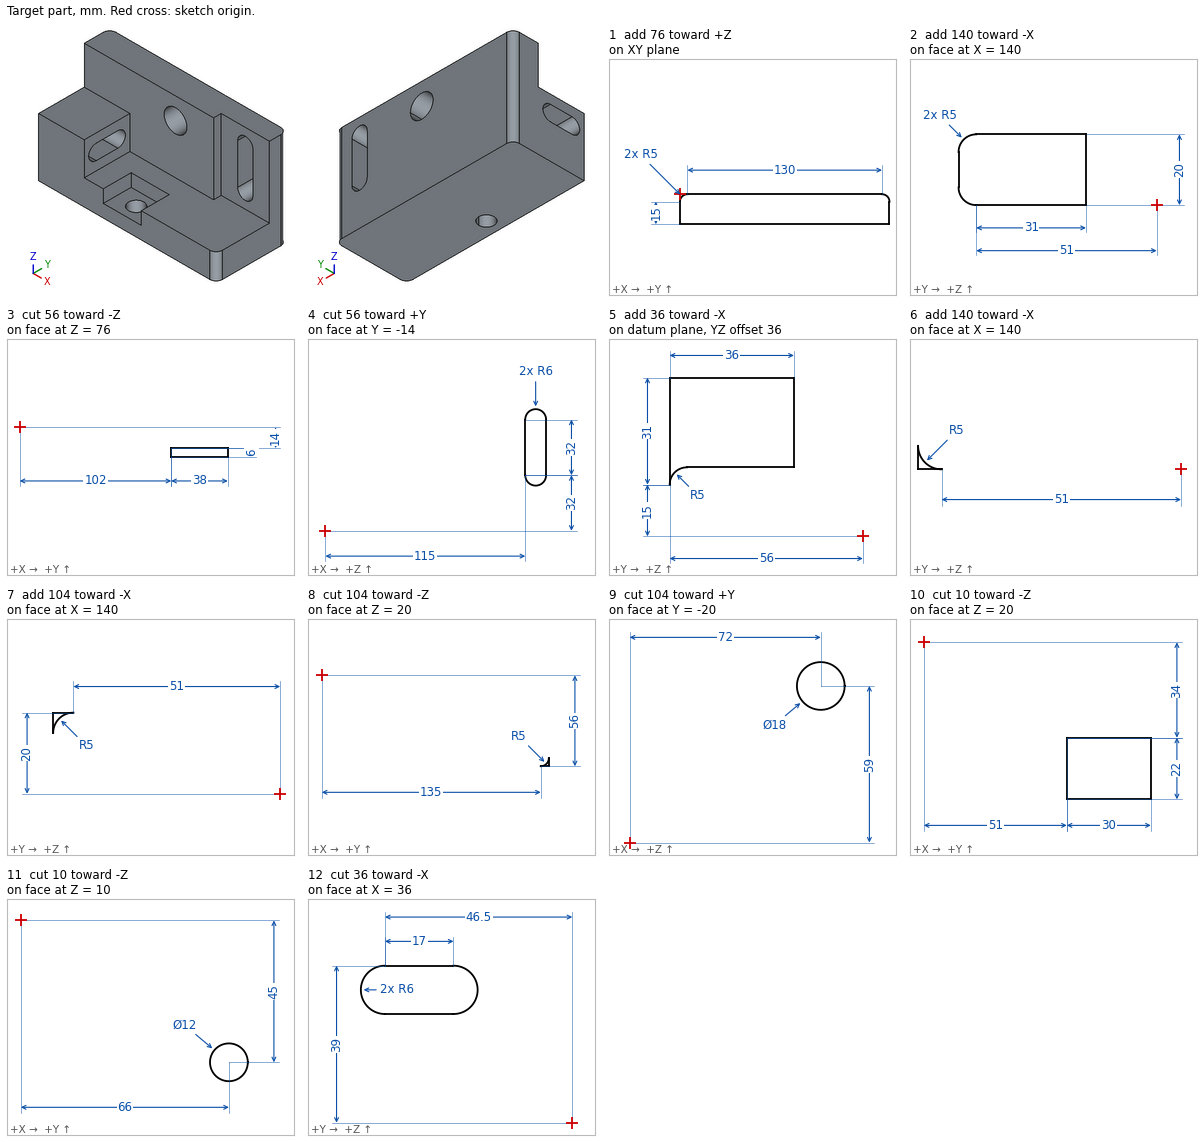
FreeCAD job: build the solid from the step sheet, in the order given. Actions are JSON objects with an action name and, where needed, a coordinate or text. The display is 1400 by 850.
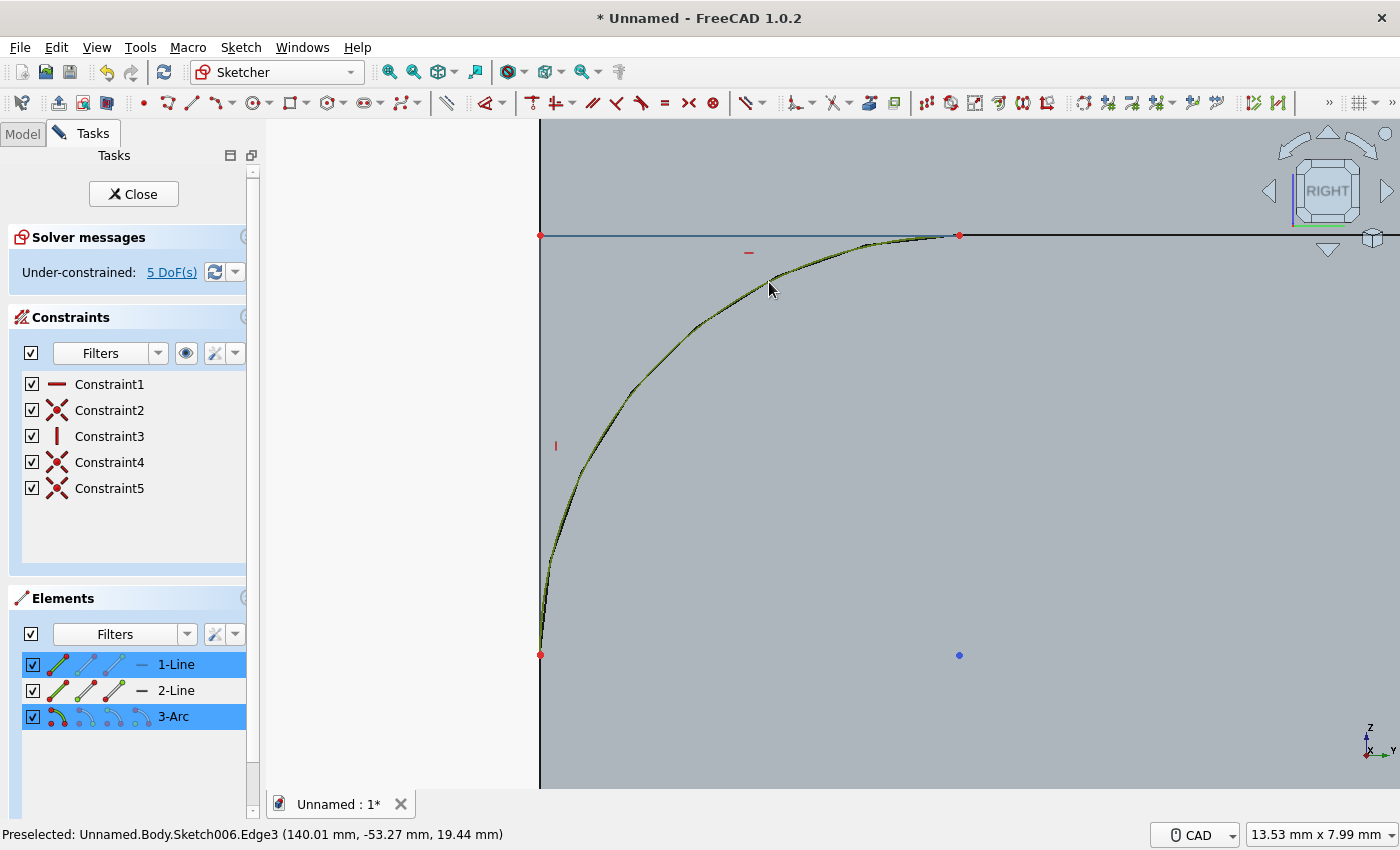
{"action": "key", "text": "t"}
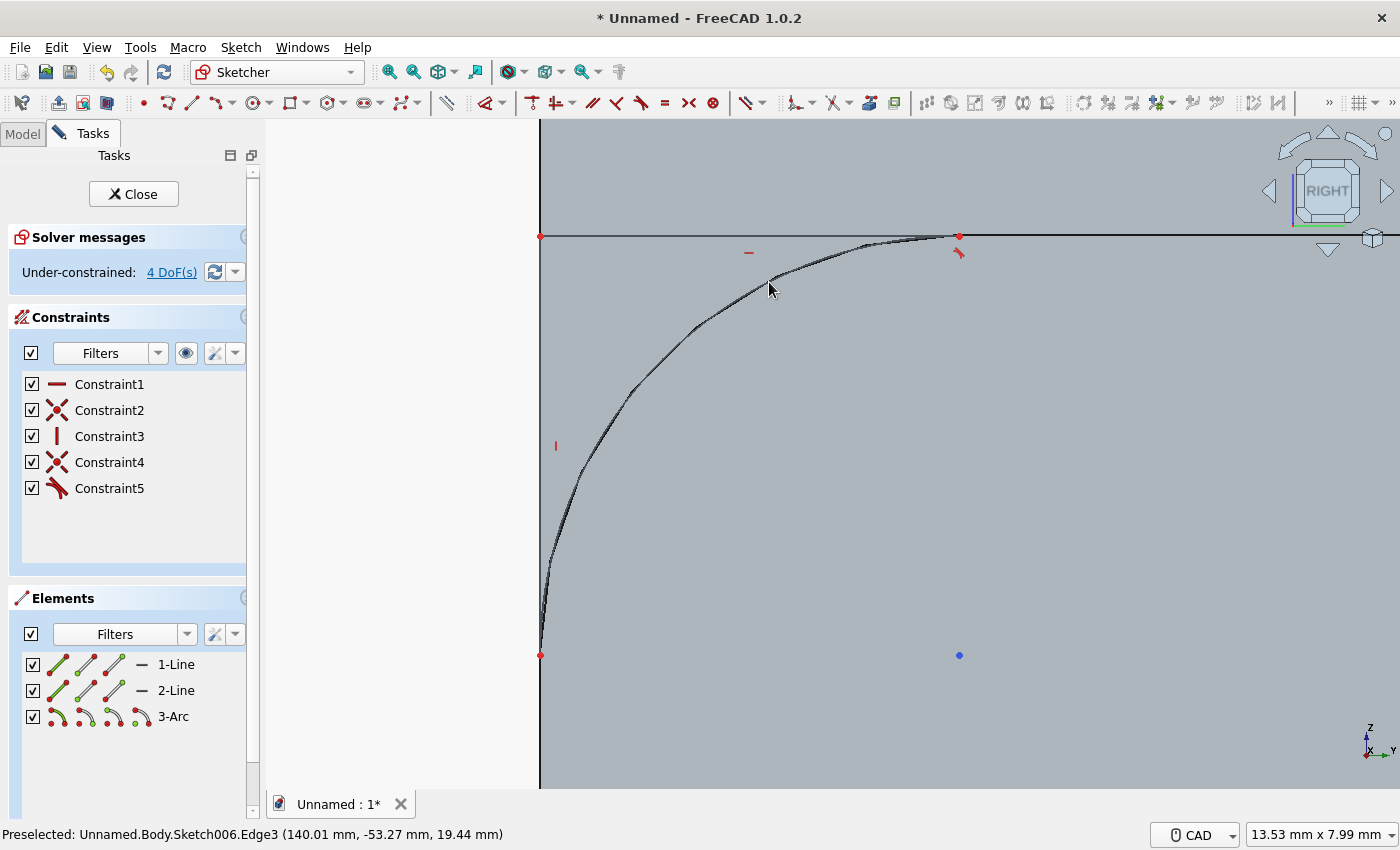
{"action": "left_click", "coordinate": [540, 362]}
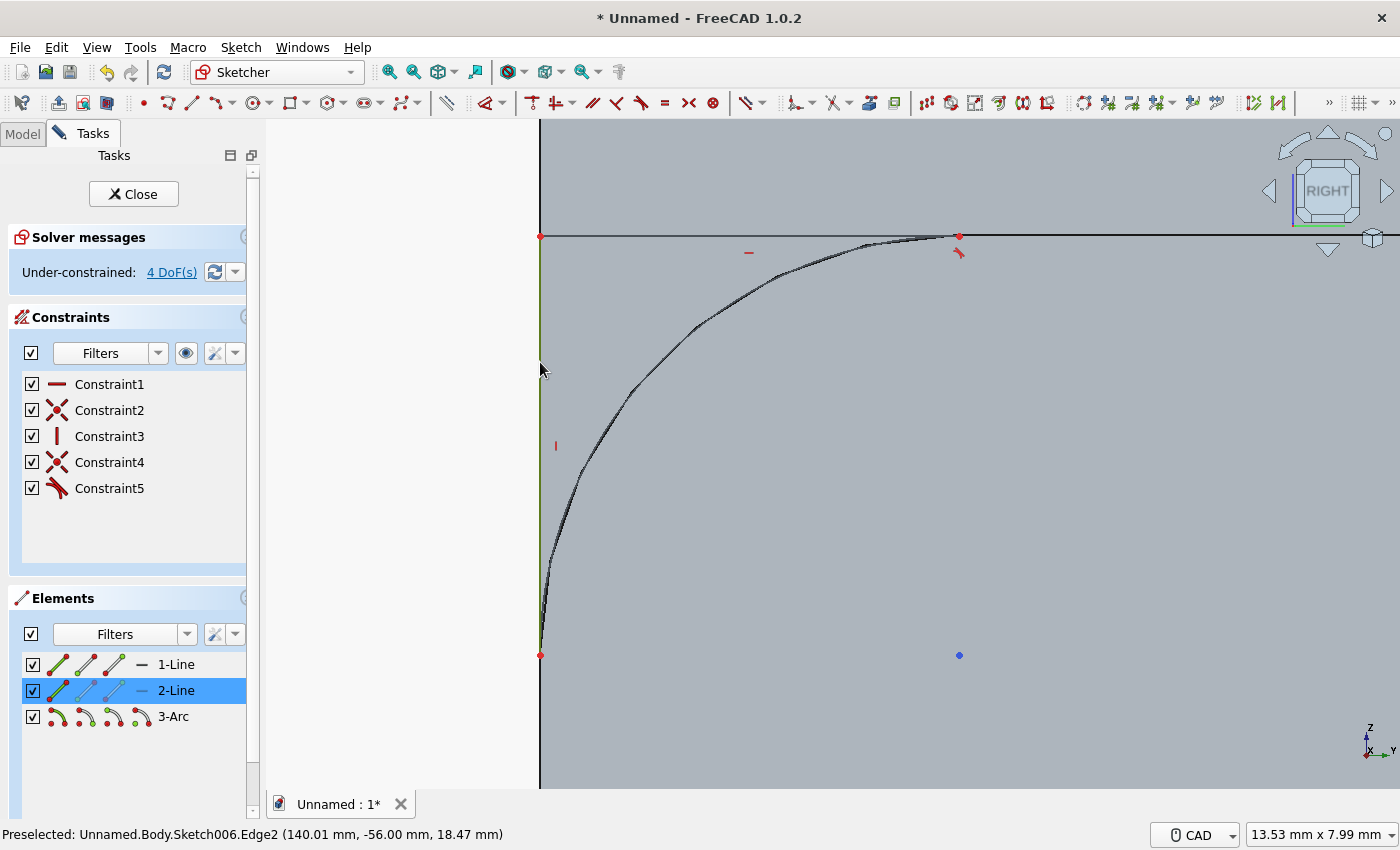
{"action": "left_click", "coordinate": [770, 282]}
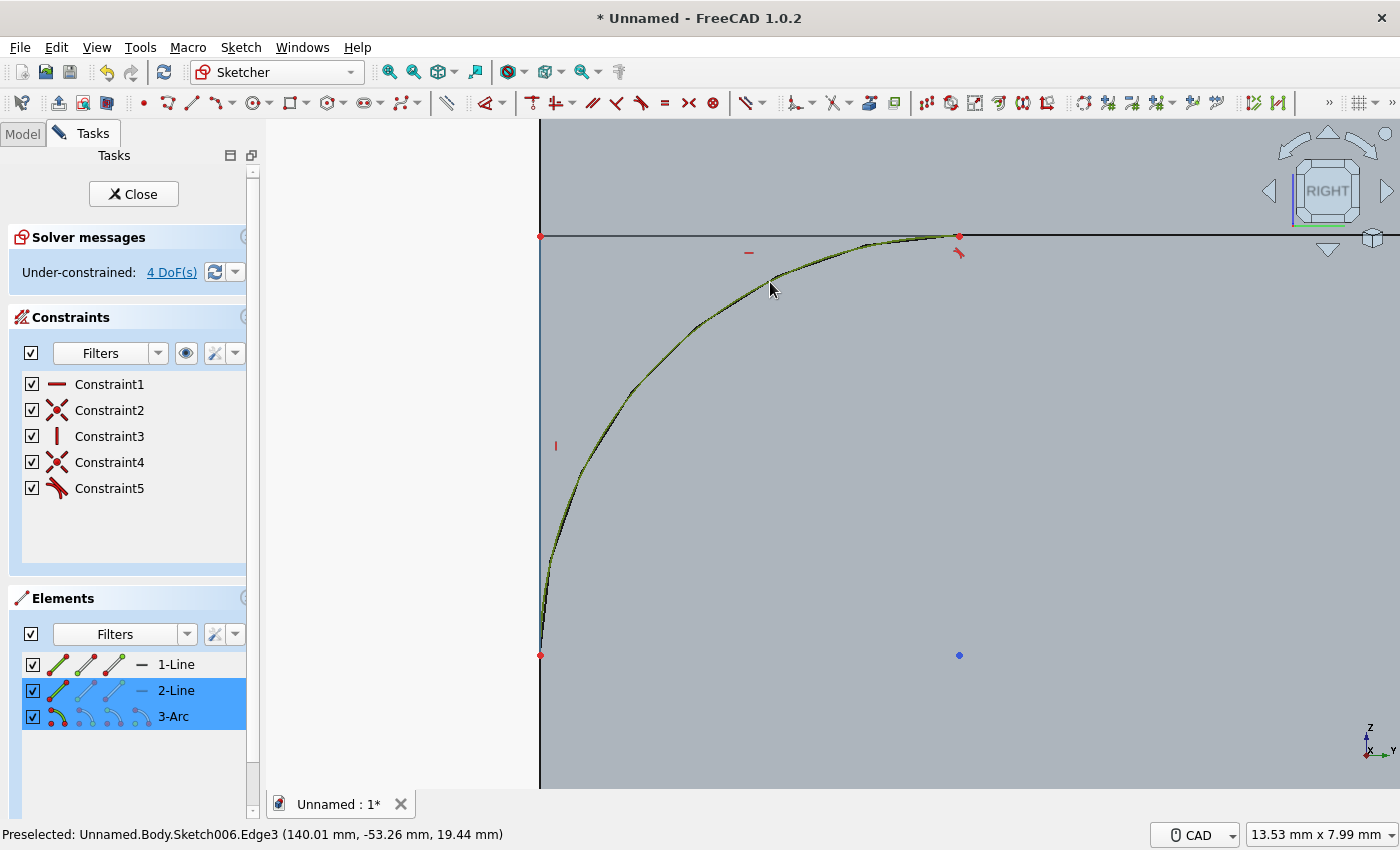
{"action": "left_click", "coordinate": [642, 104]}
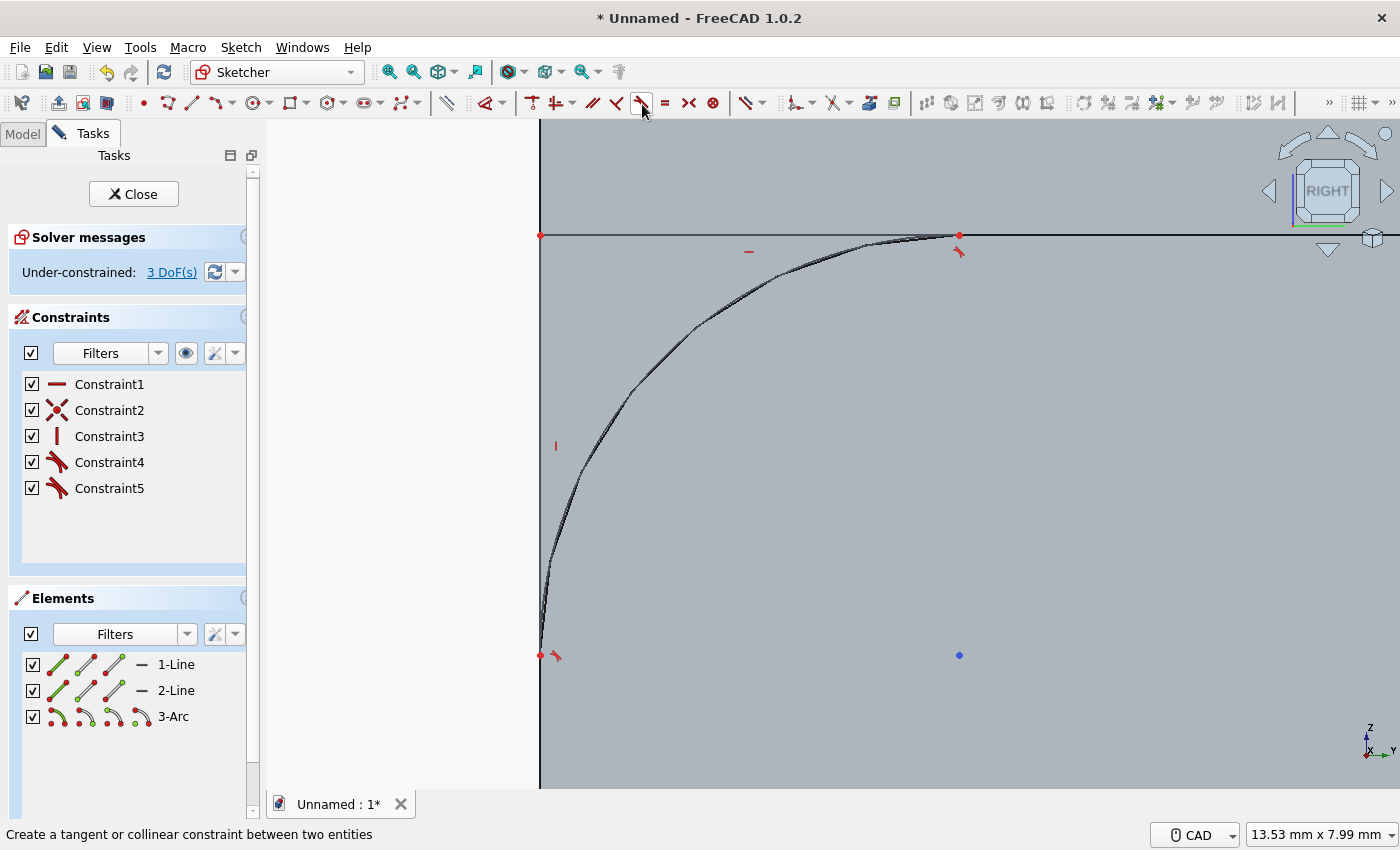
{"action": "left_click", "coordinate": [486, 104]}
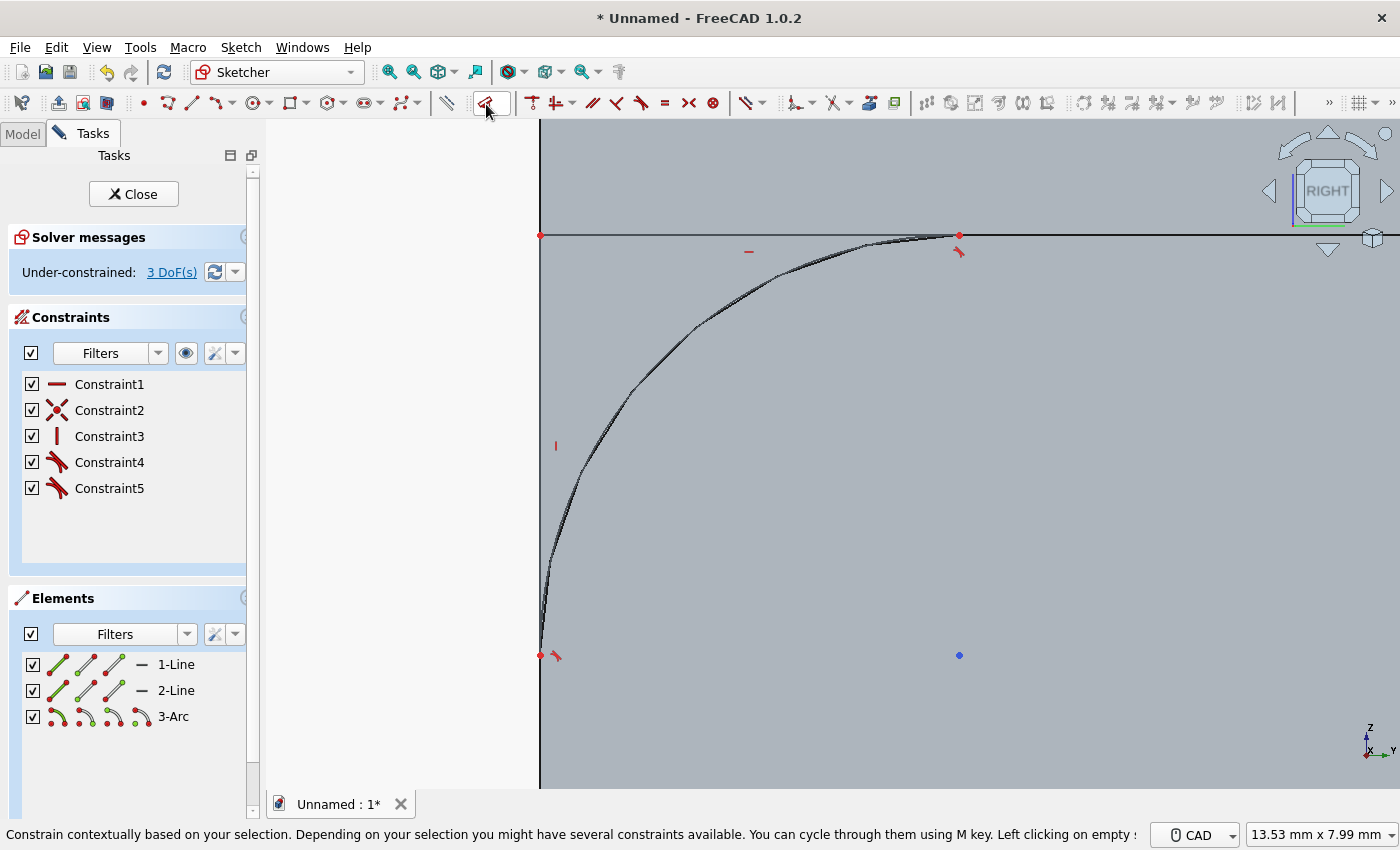
{"action": "left_click", "coordinate": [769, 281]}
{"action": "left_click", "coordinate": [754, 252]}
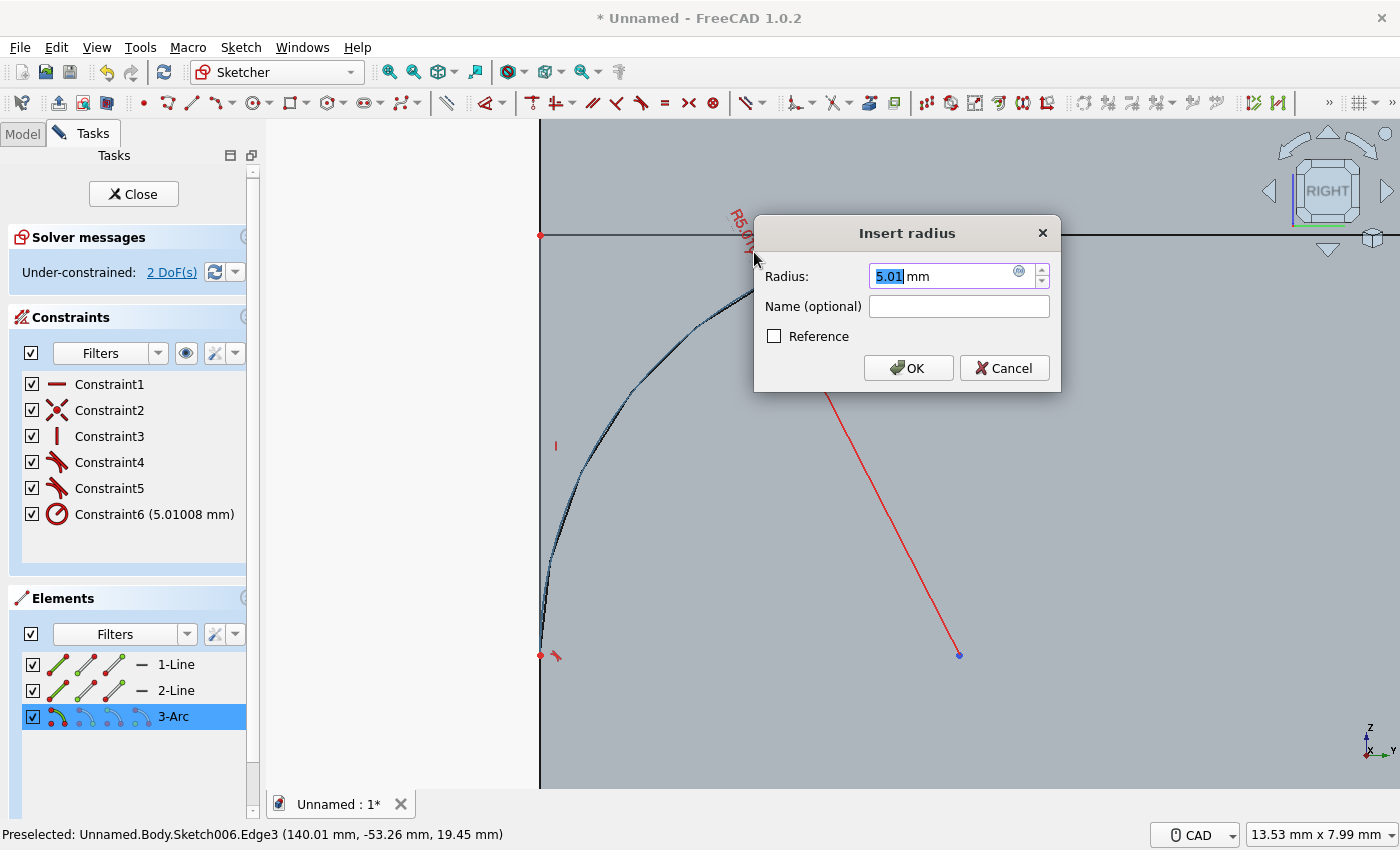
{"action": "type", "text": "5"}
{"action": "key", "text": "Return"}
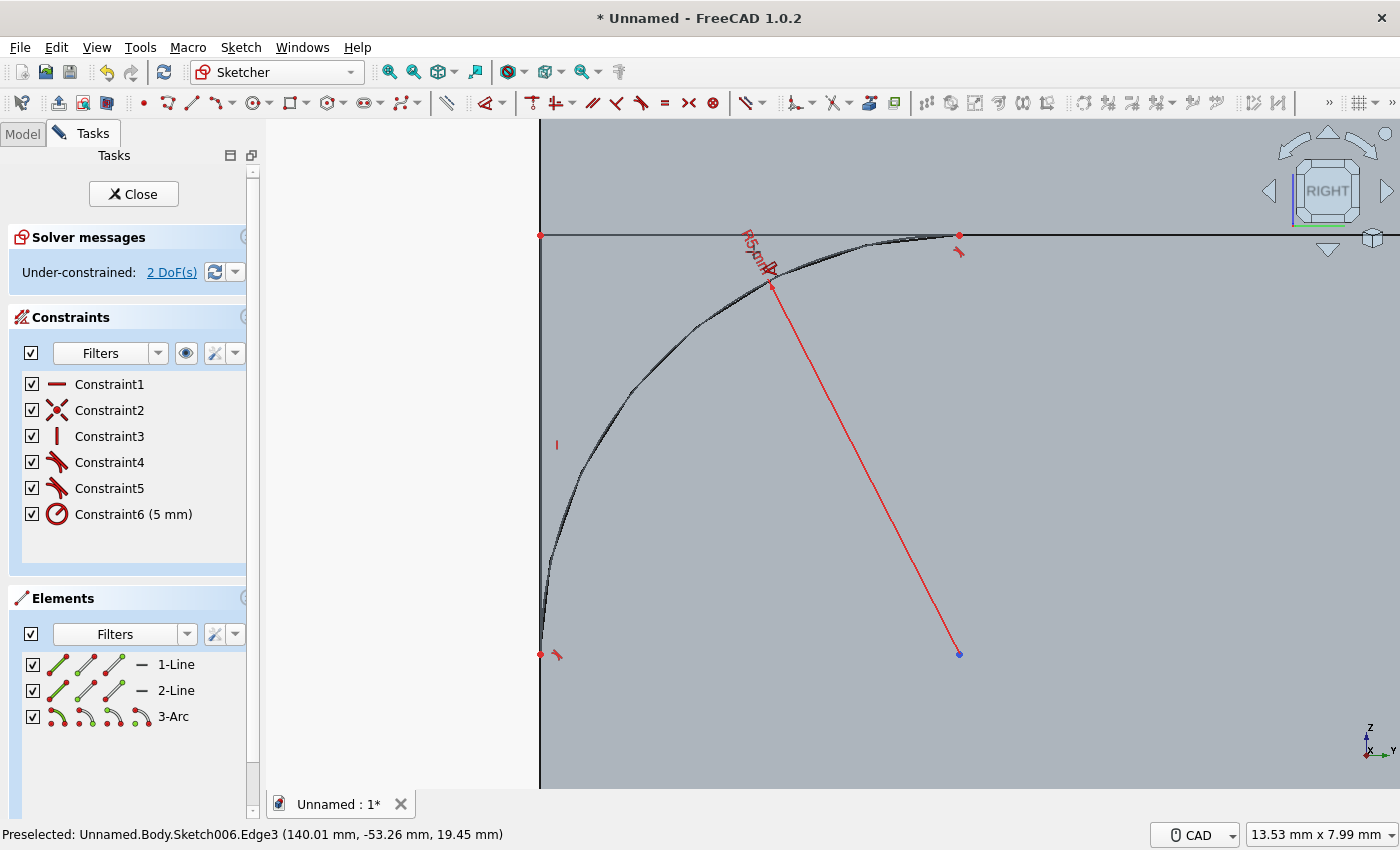
{"action": "left_click", "coordinate": [960, 235]}
{"action": "left_click", "coordinate": [1097, 201]}